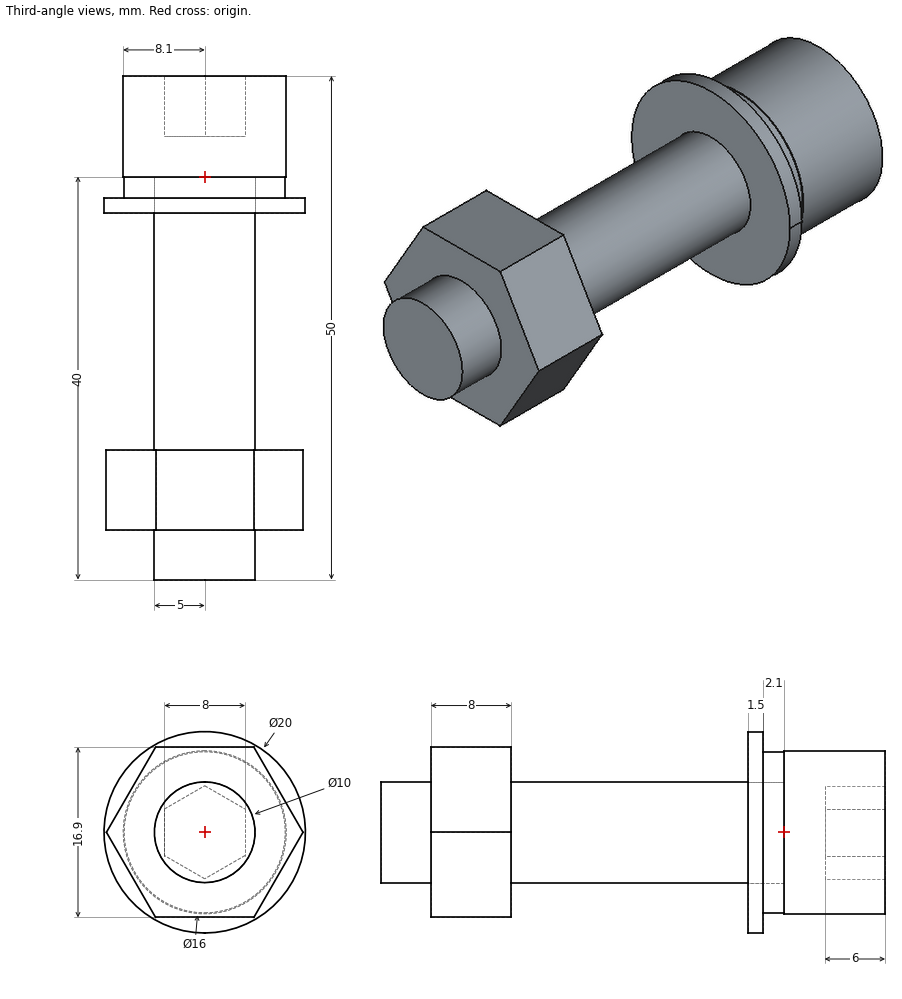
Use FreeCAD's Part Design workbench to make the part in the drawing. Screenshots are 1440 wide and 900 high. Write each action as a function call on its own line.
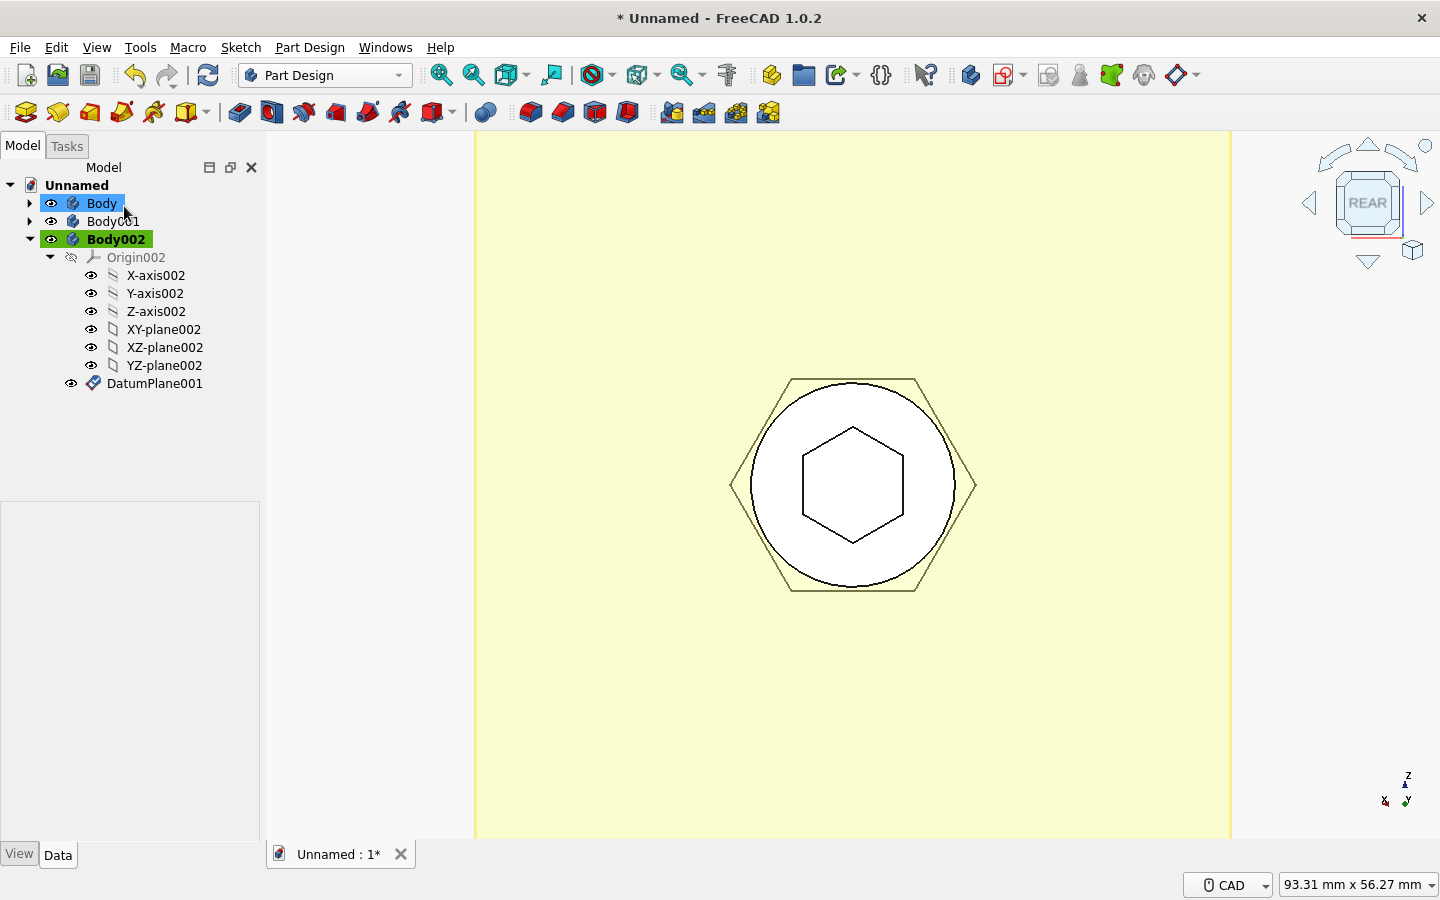
click(116, 383)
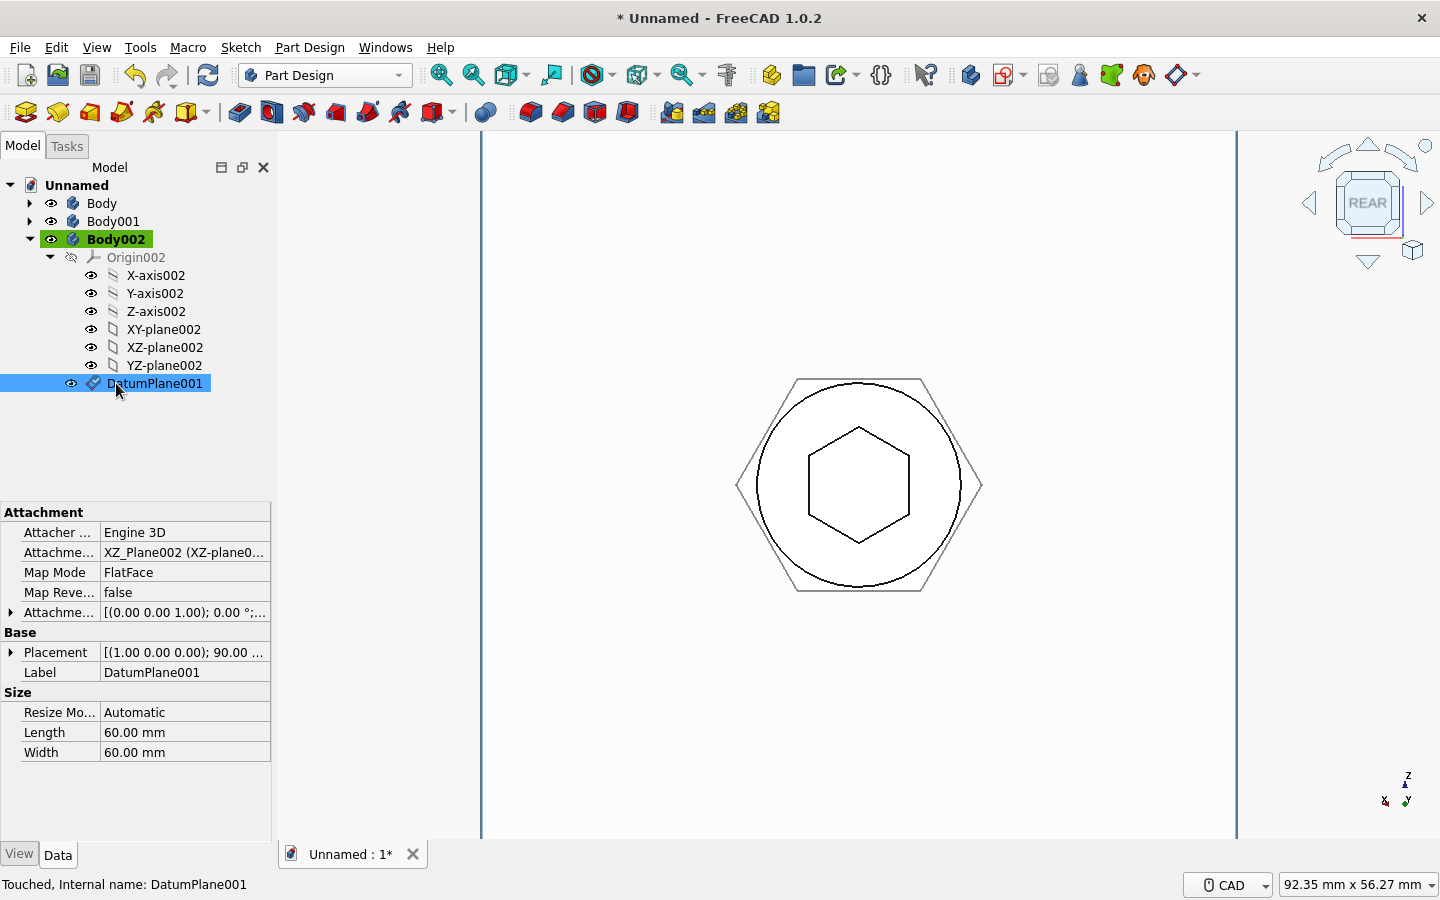
click(1004, 76)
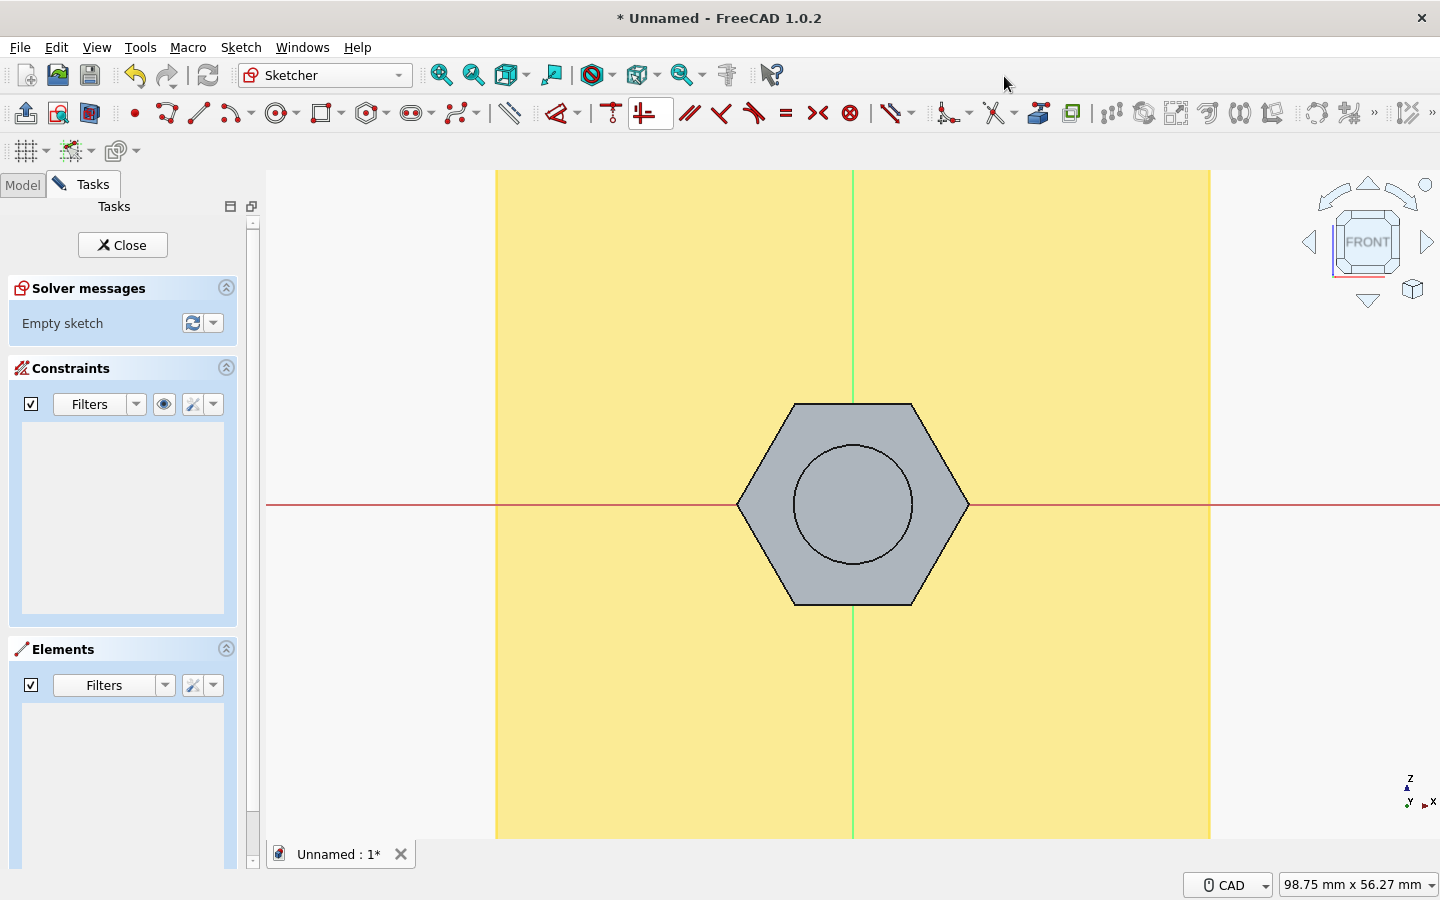
scroll(936, 505, up, 3)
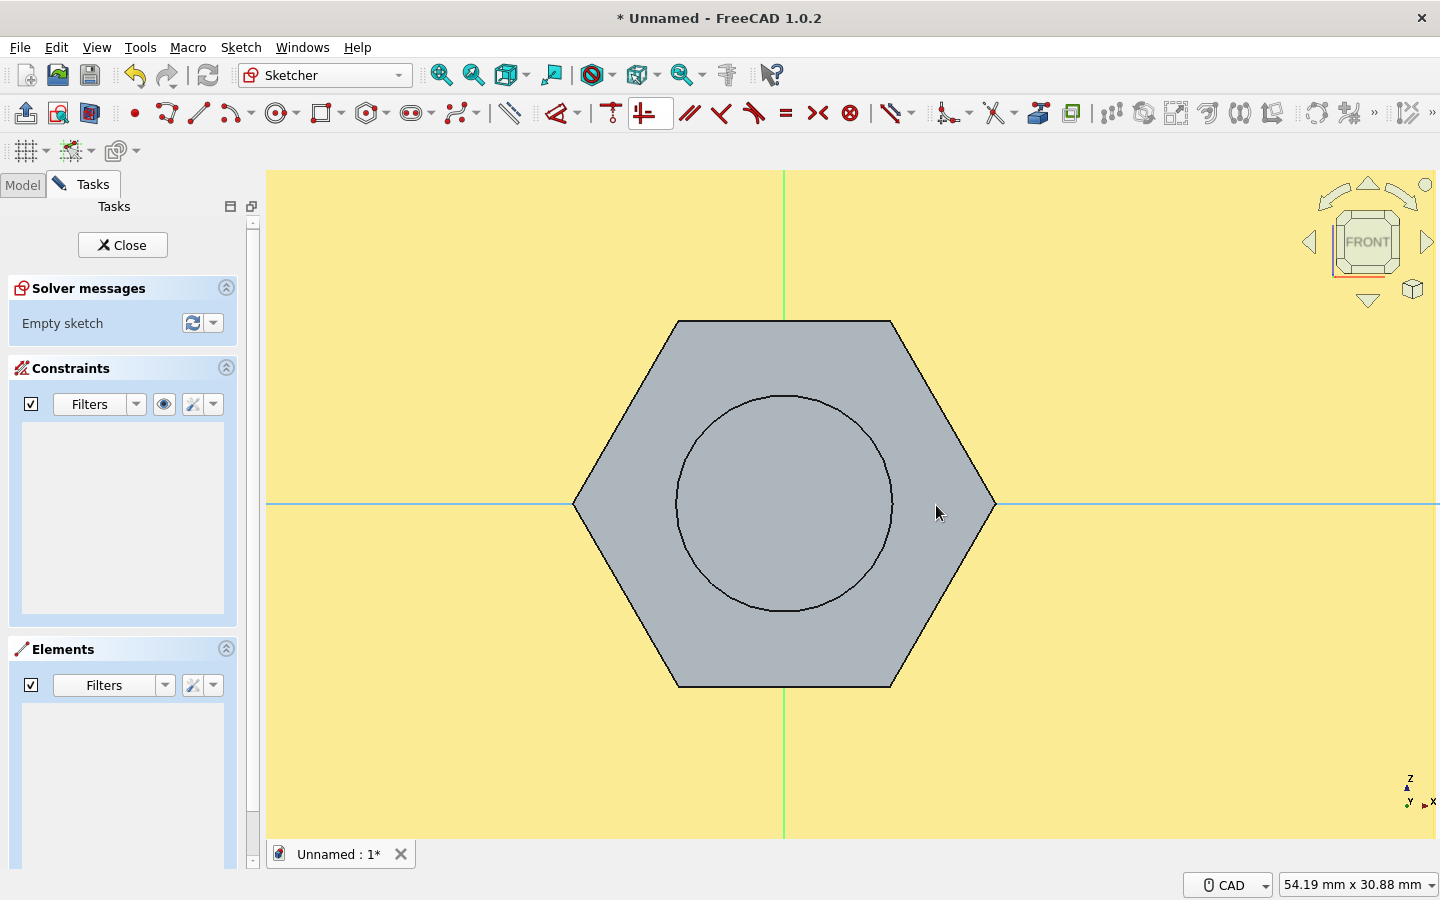
click(276, 114)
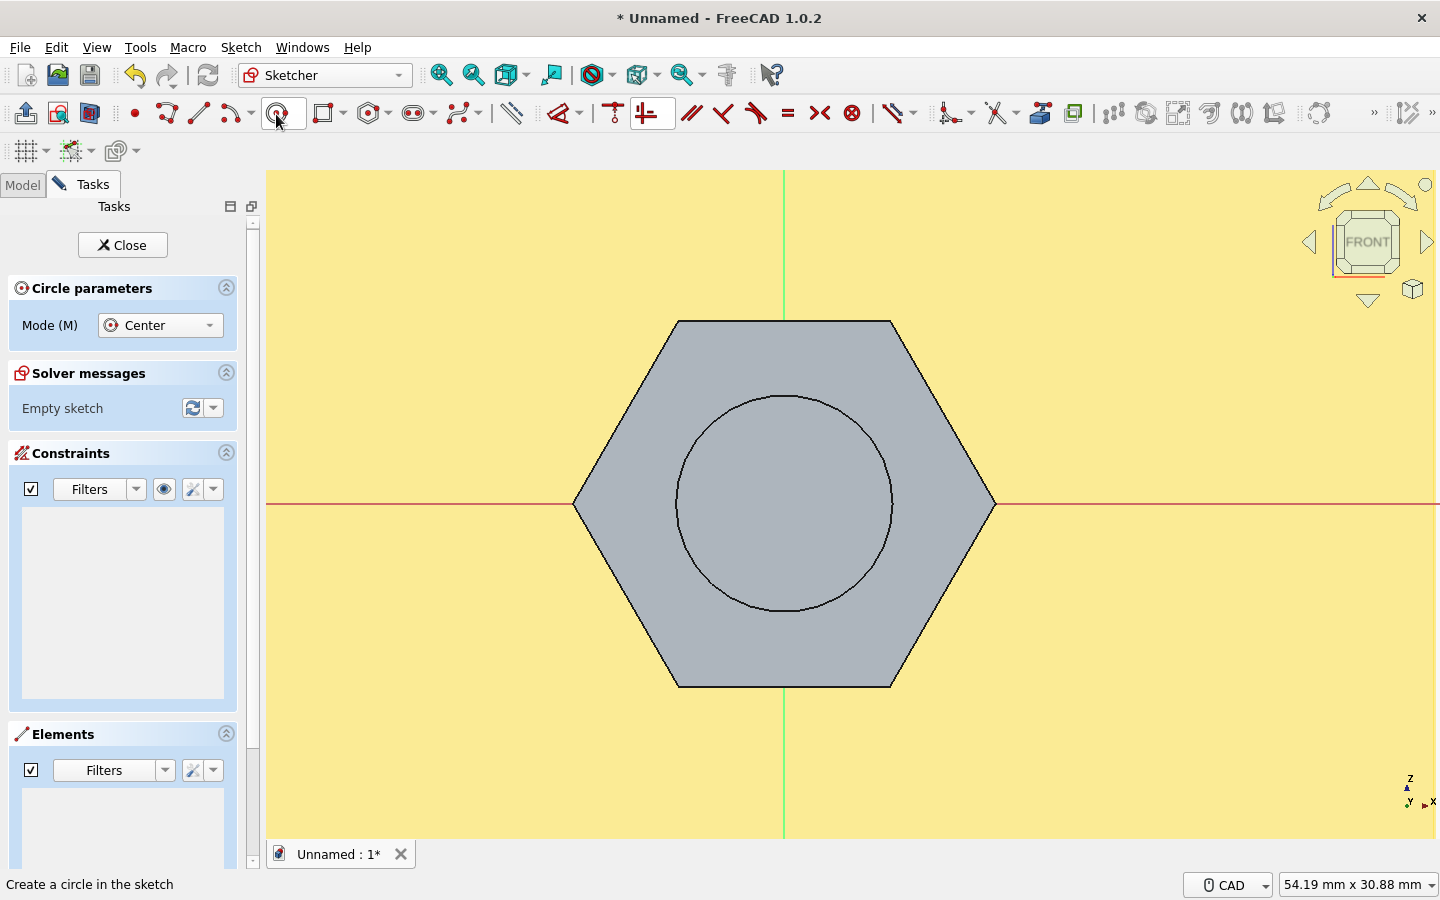
click(784, 504)
move(937, 350)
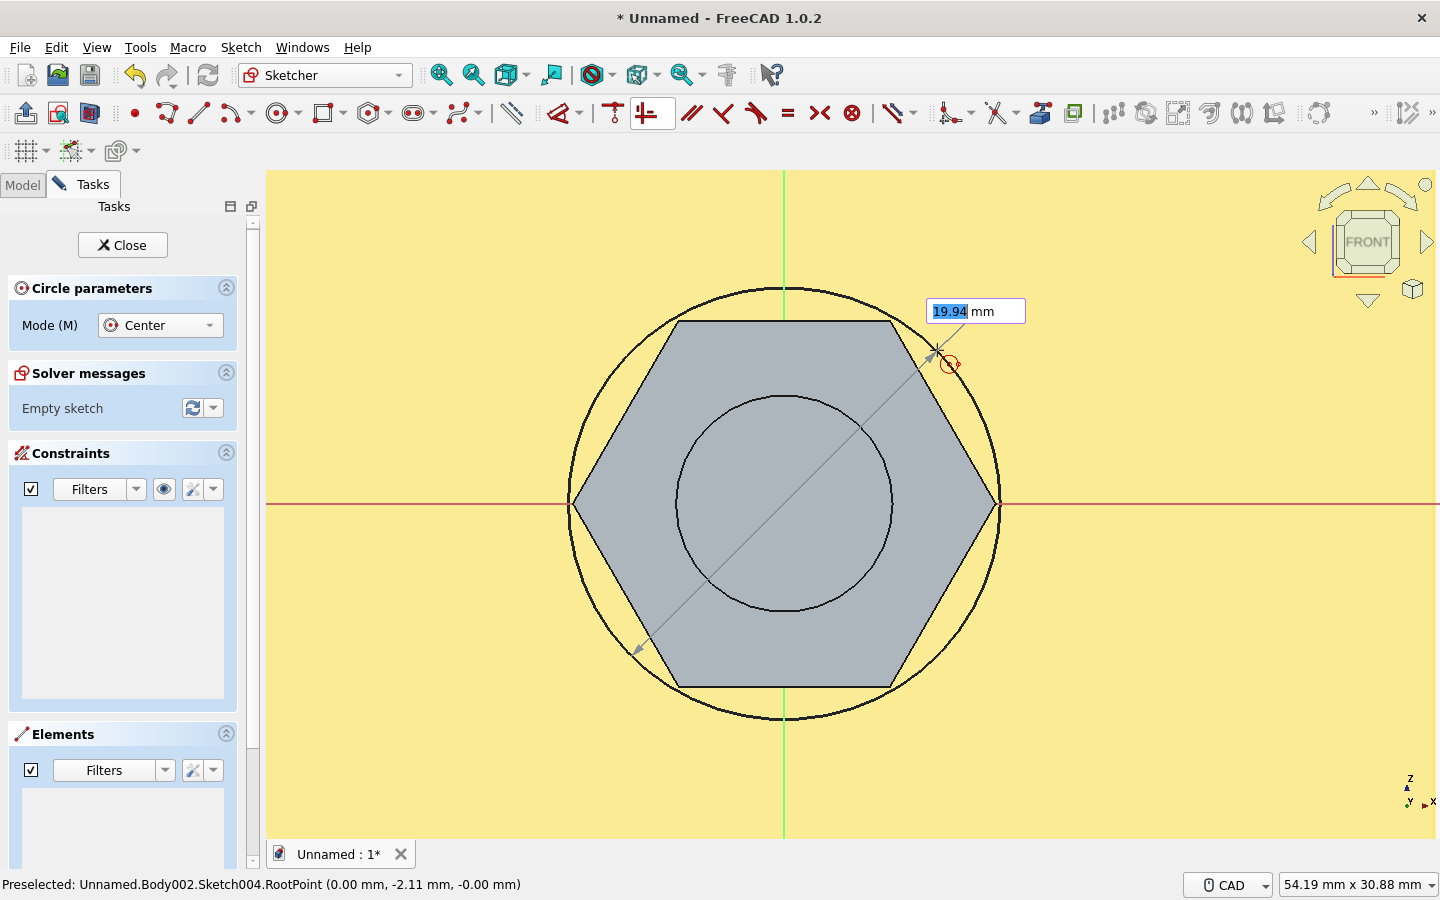
text(20)
key(Return)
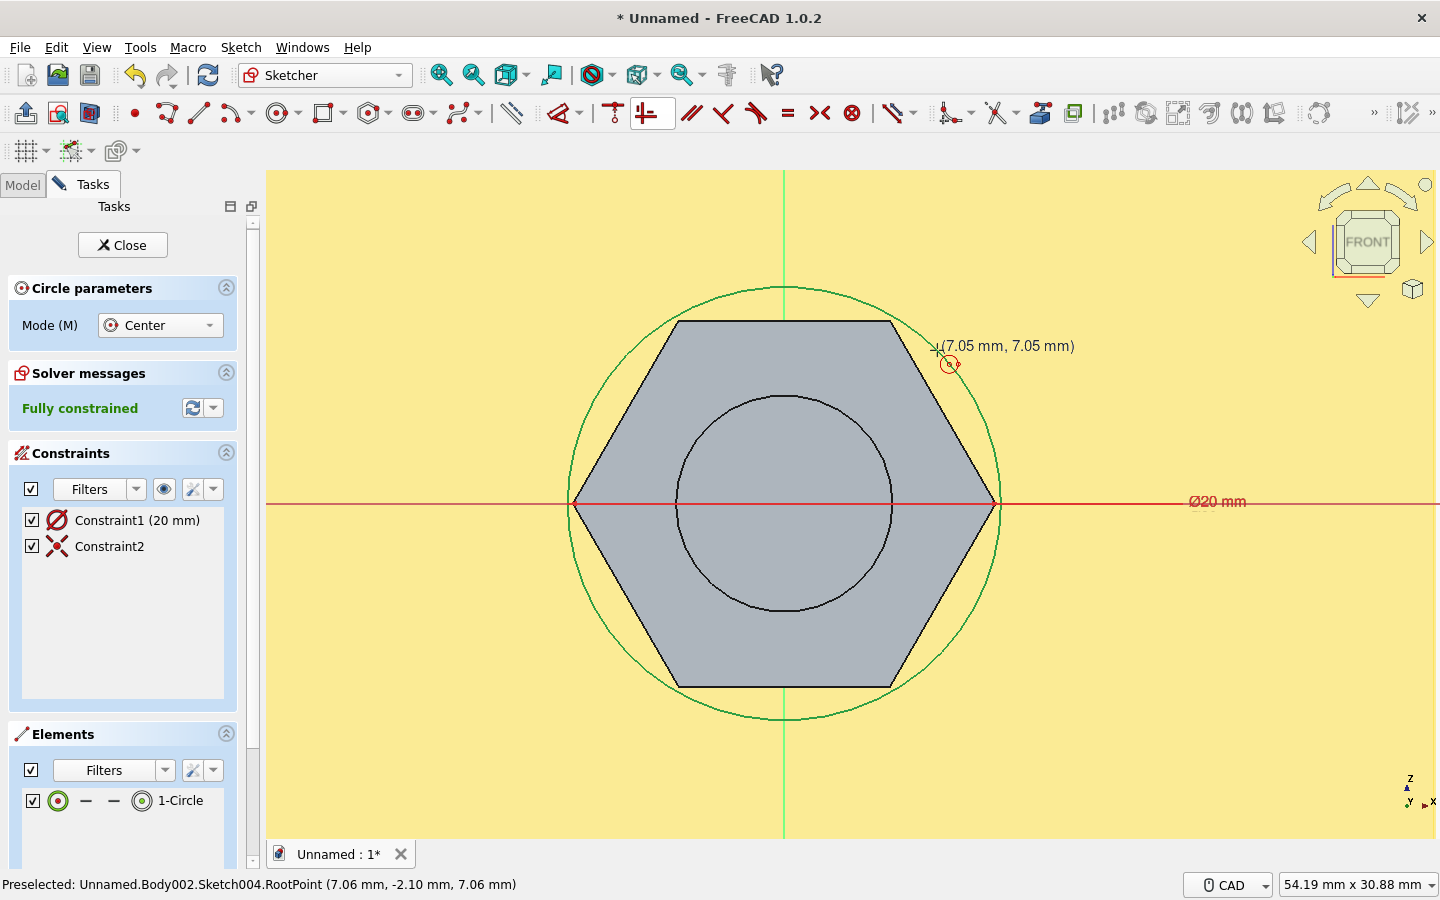
click(784, 504)
move(861, 427)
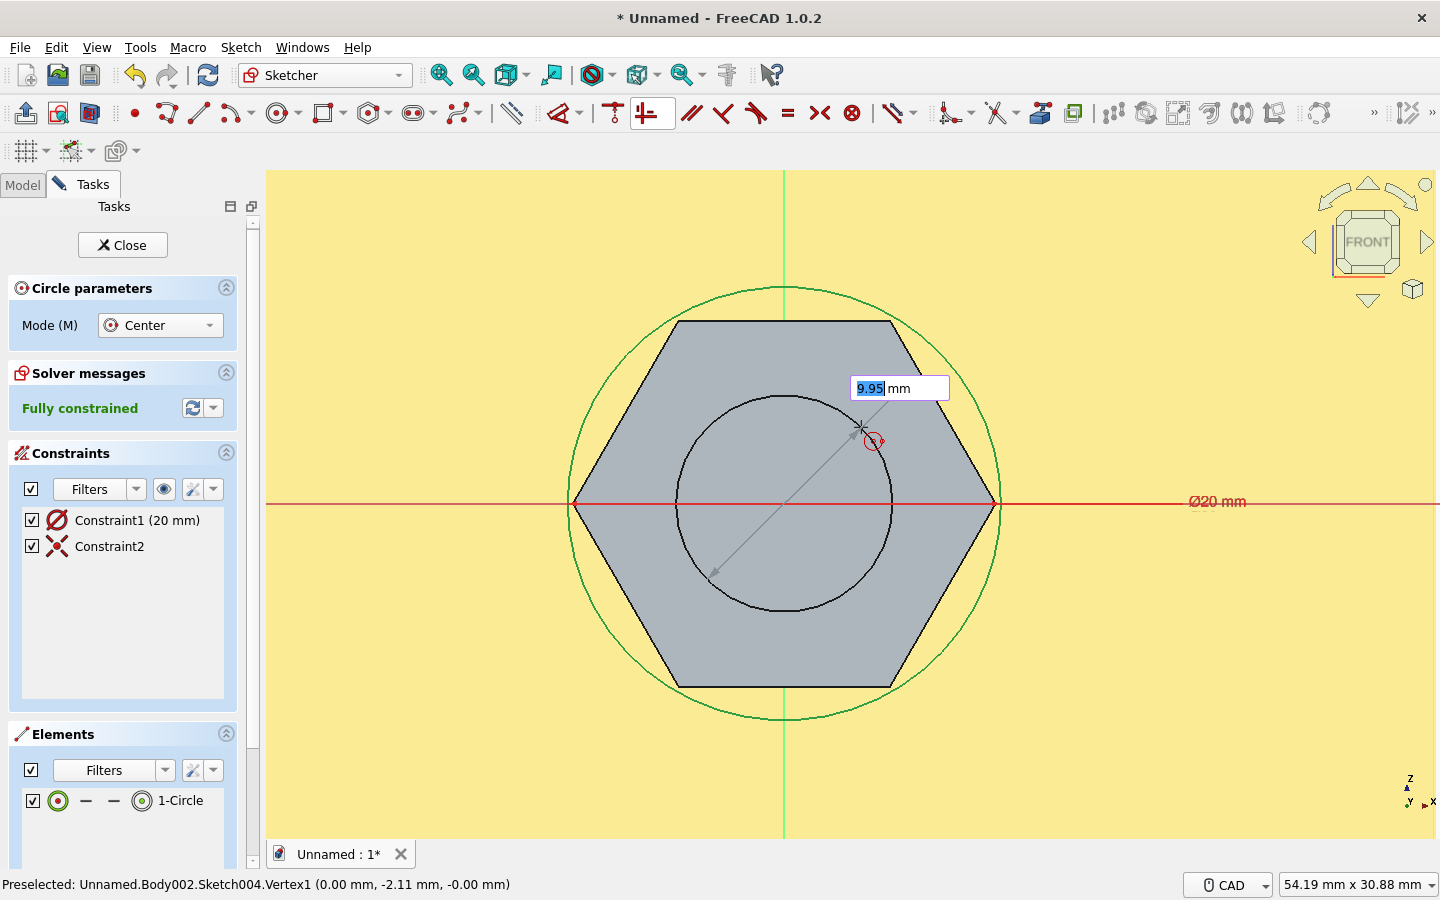
text(10)
key(Return)
key(Escape)